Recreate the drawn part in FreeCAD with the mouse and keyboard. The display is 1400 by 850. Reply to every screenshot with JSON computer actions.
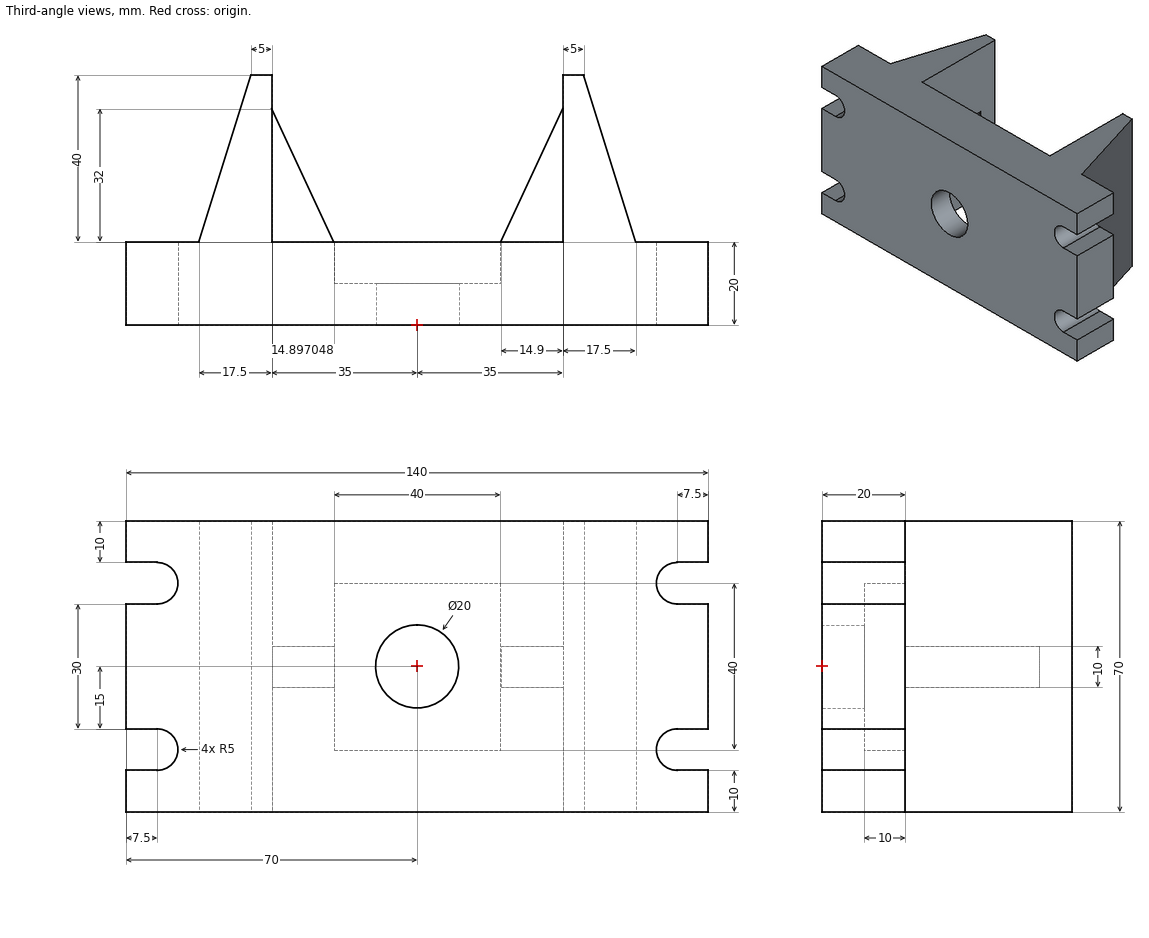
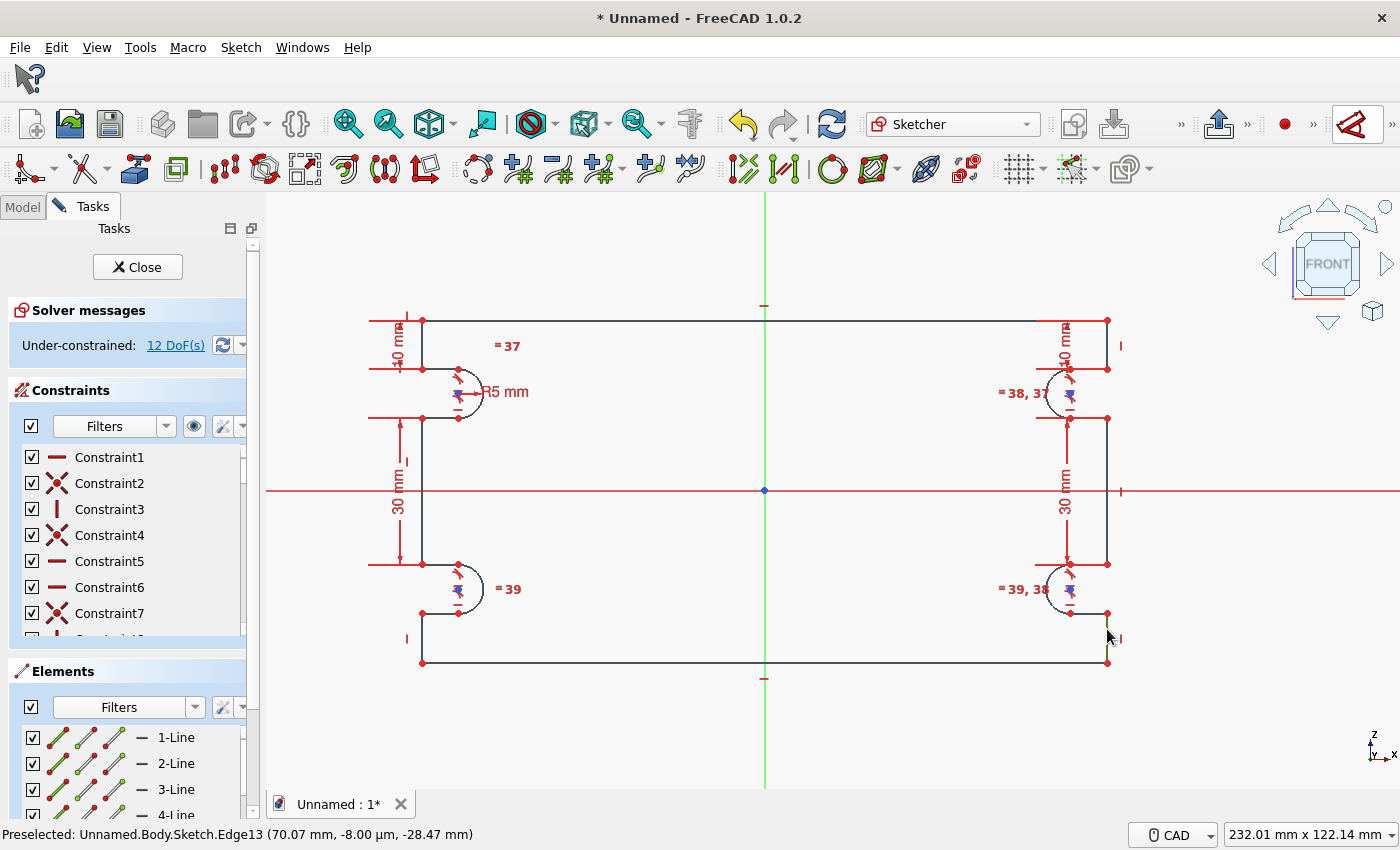
{"action": "key", "text": "i"}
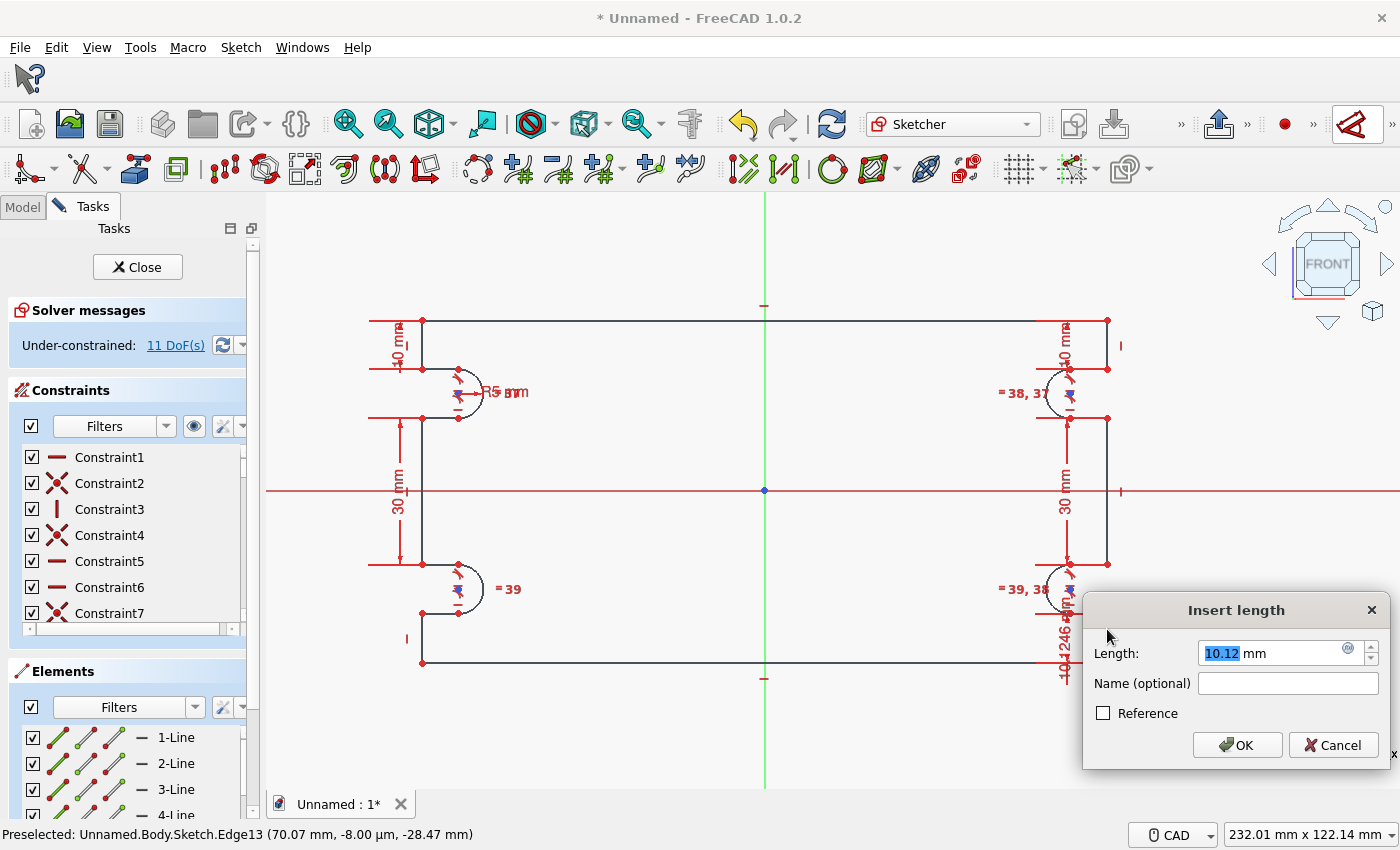
{"action": "type", "text": "10"}
{"action": "key", "text": "Return"}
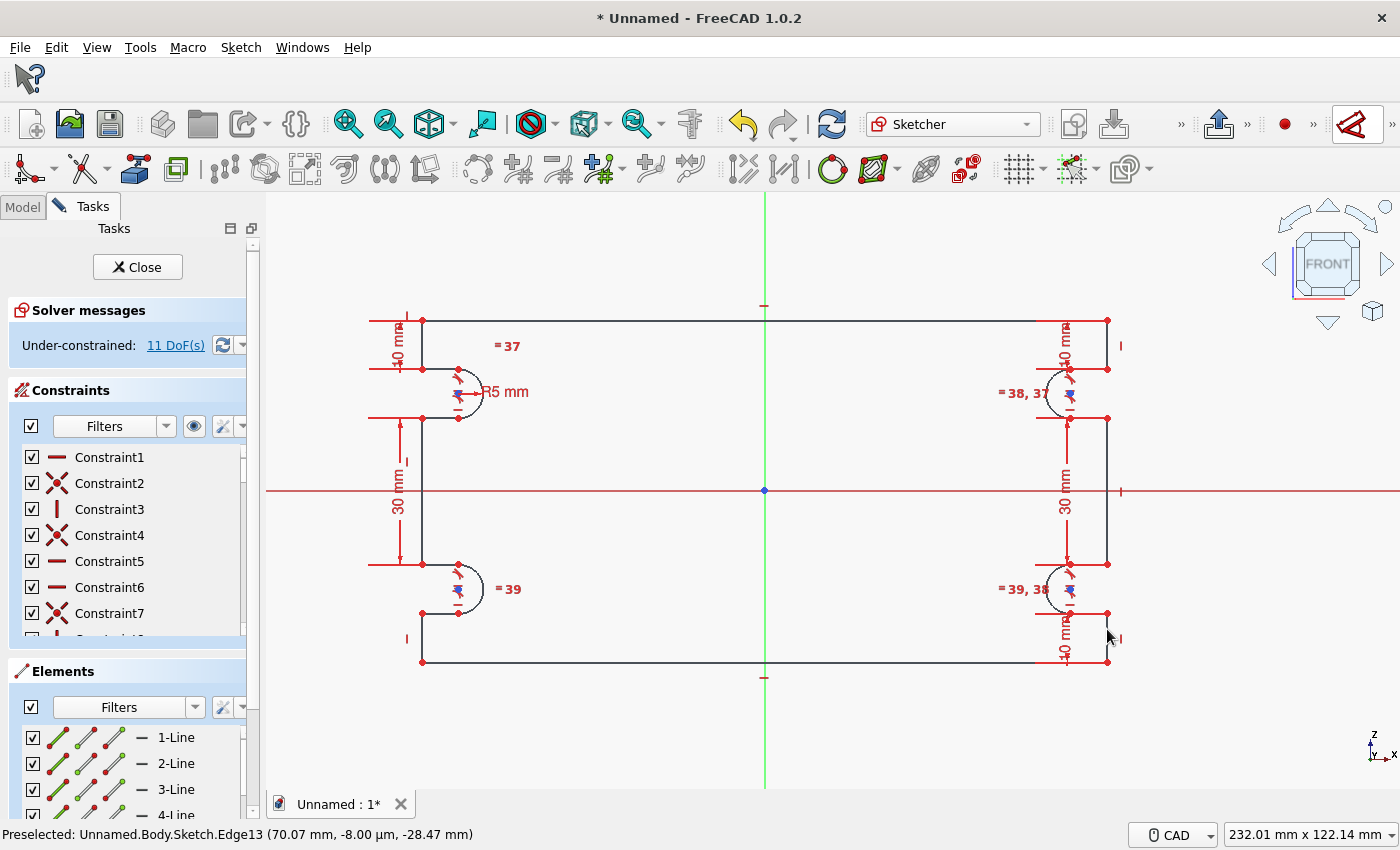
{"action": "scroll", "coordinate": [448, 565], "scroll_direction": "up", "scroll_amount": 2}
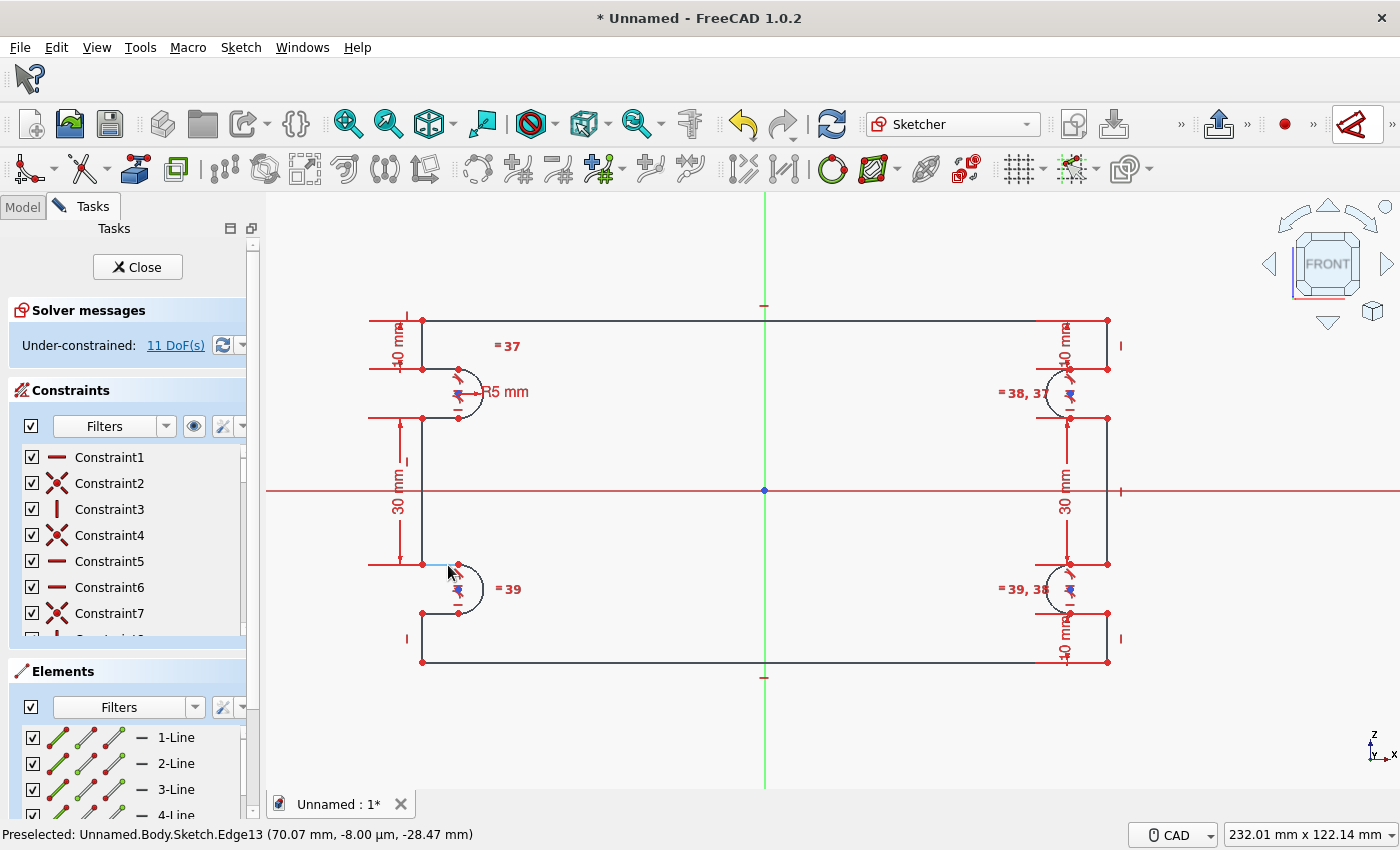
{"action": "left_click", "coordinate": [448, 565]}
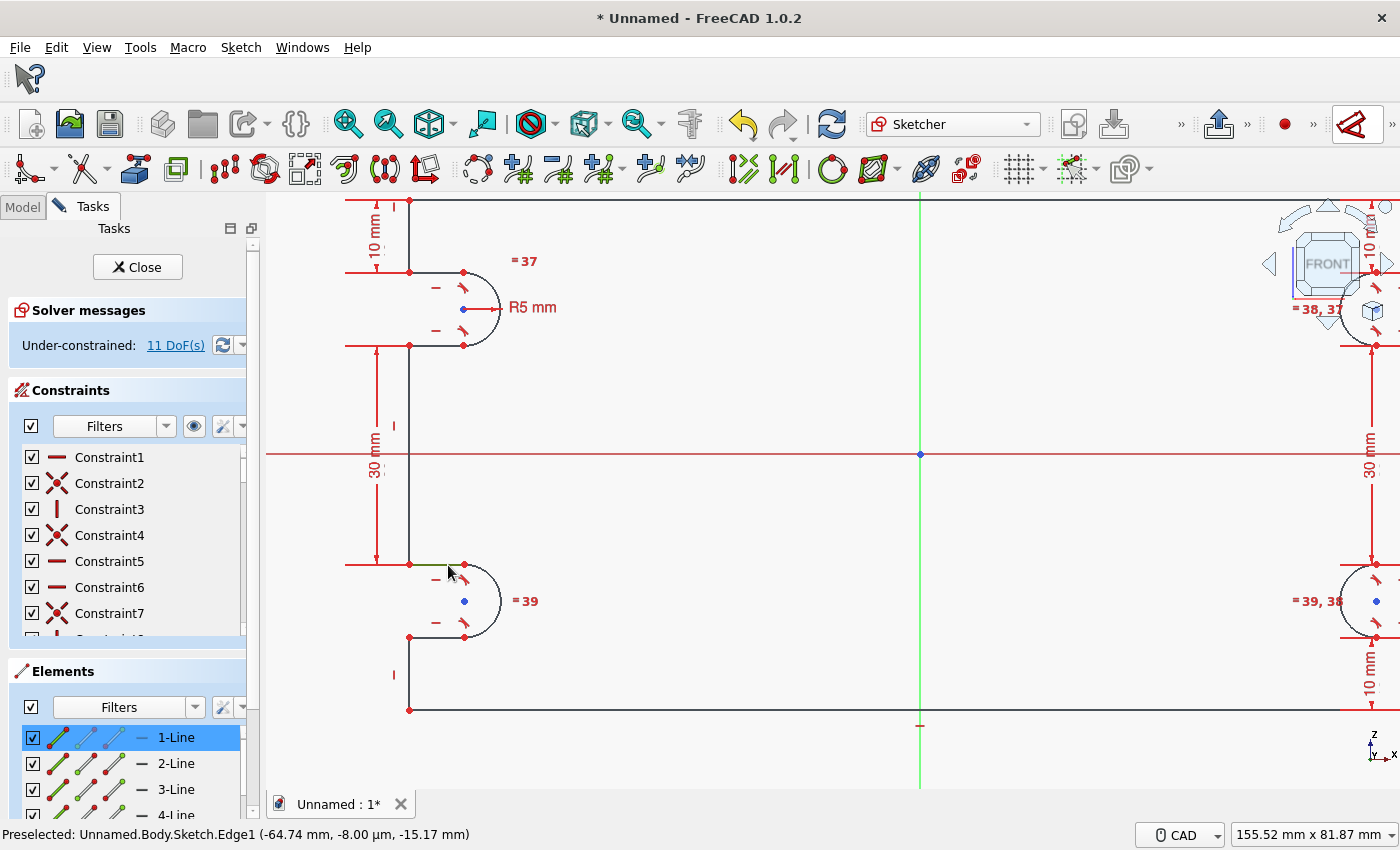
{"action": "key", "text": "l"}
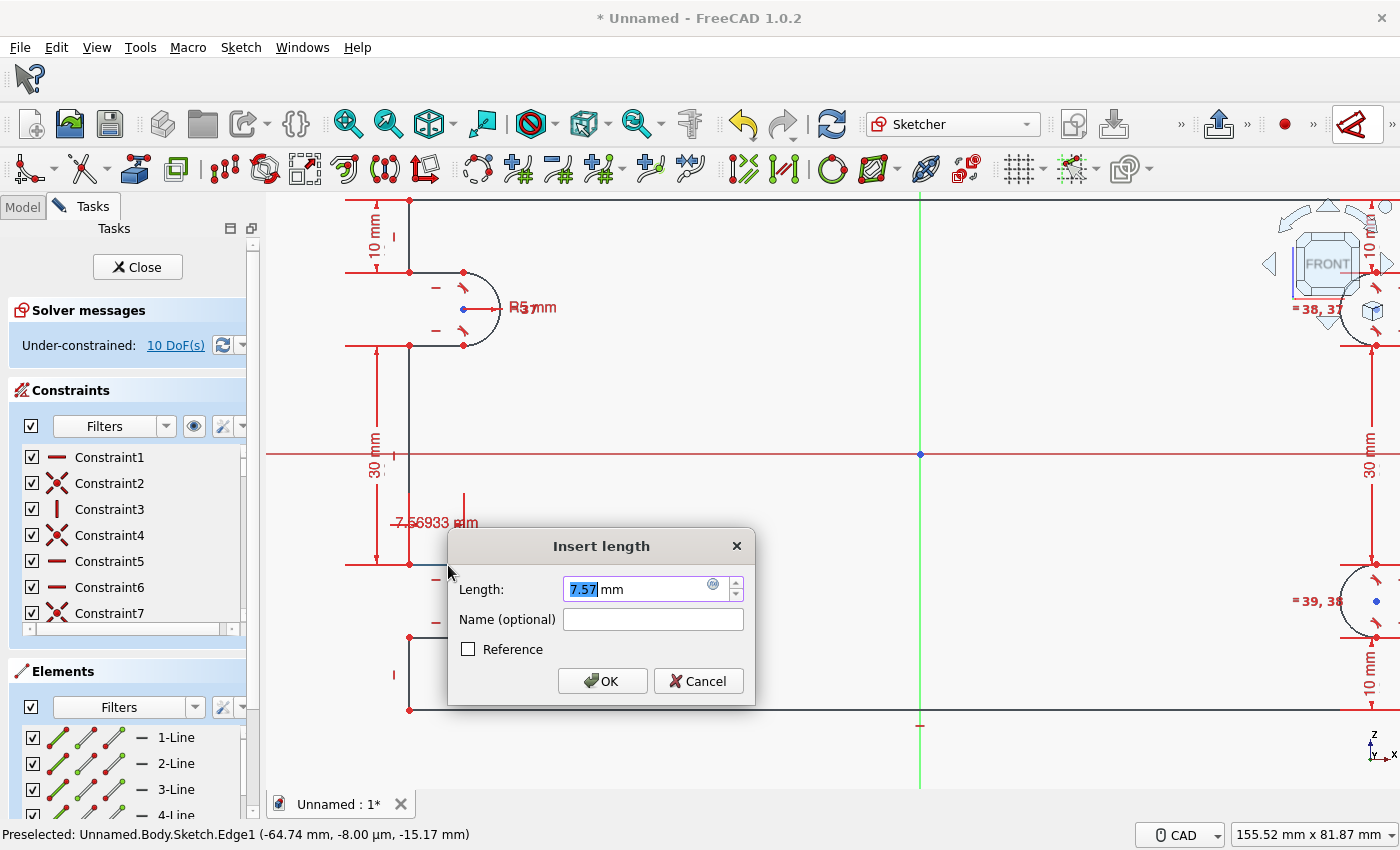
{"action": "type", "text": "7.5"}
{"action": "key", "text": "Return"}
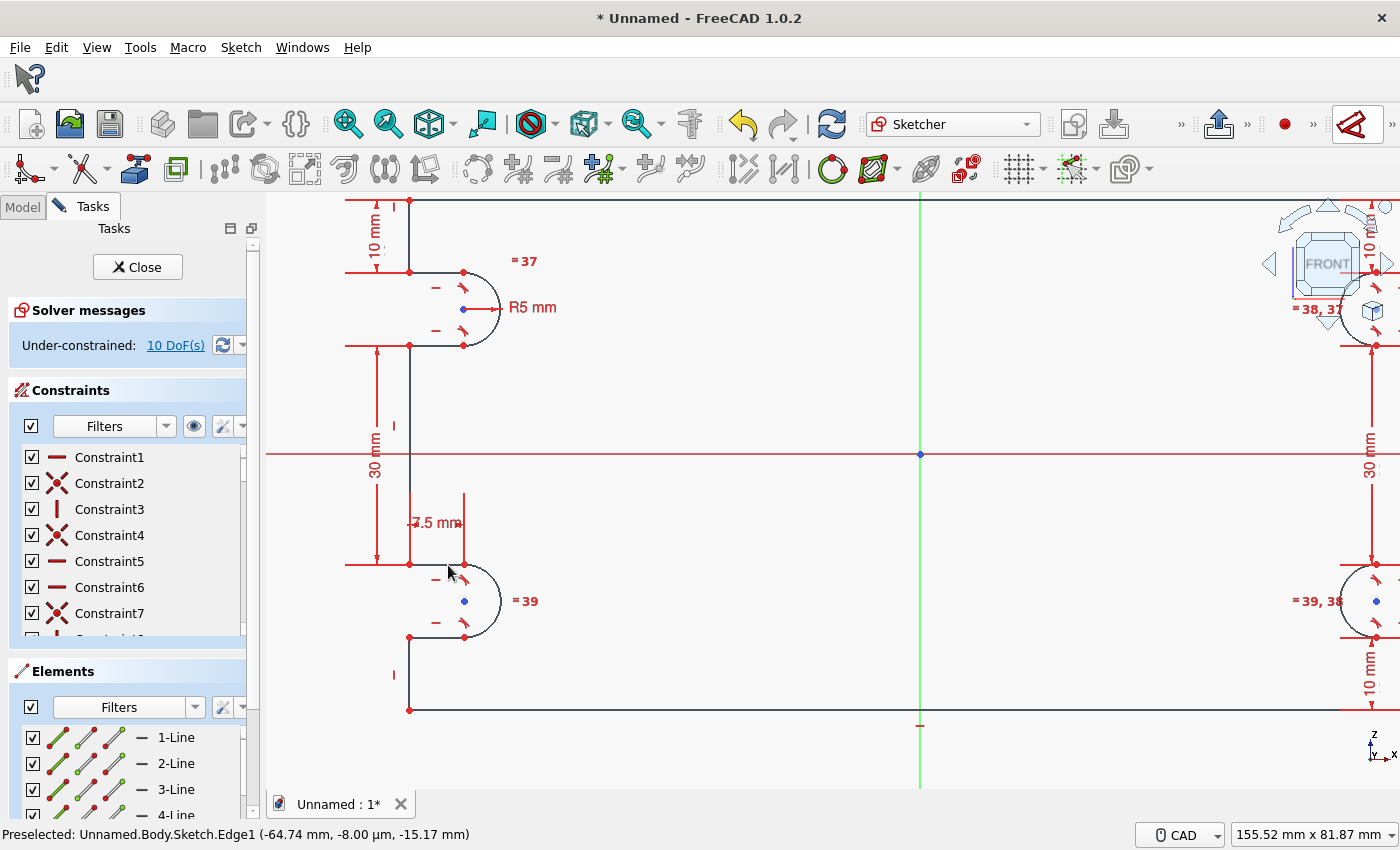
{"action": "left_click", "coordinate": [426, 346]}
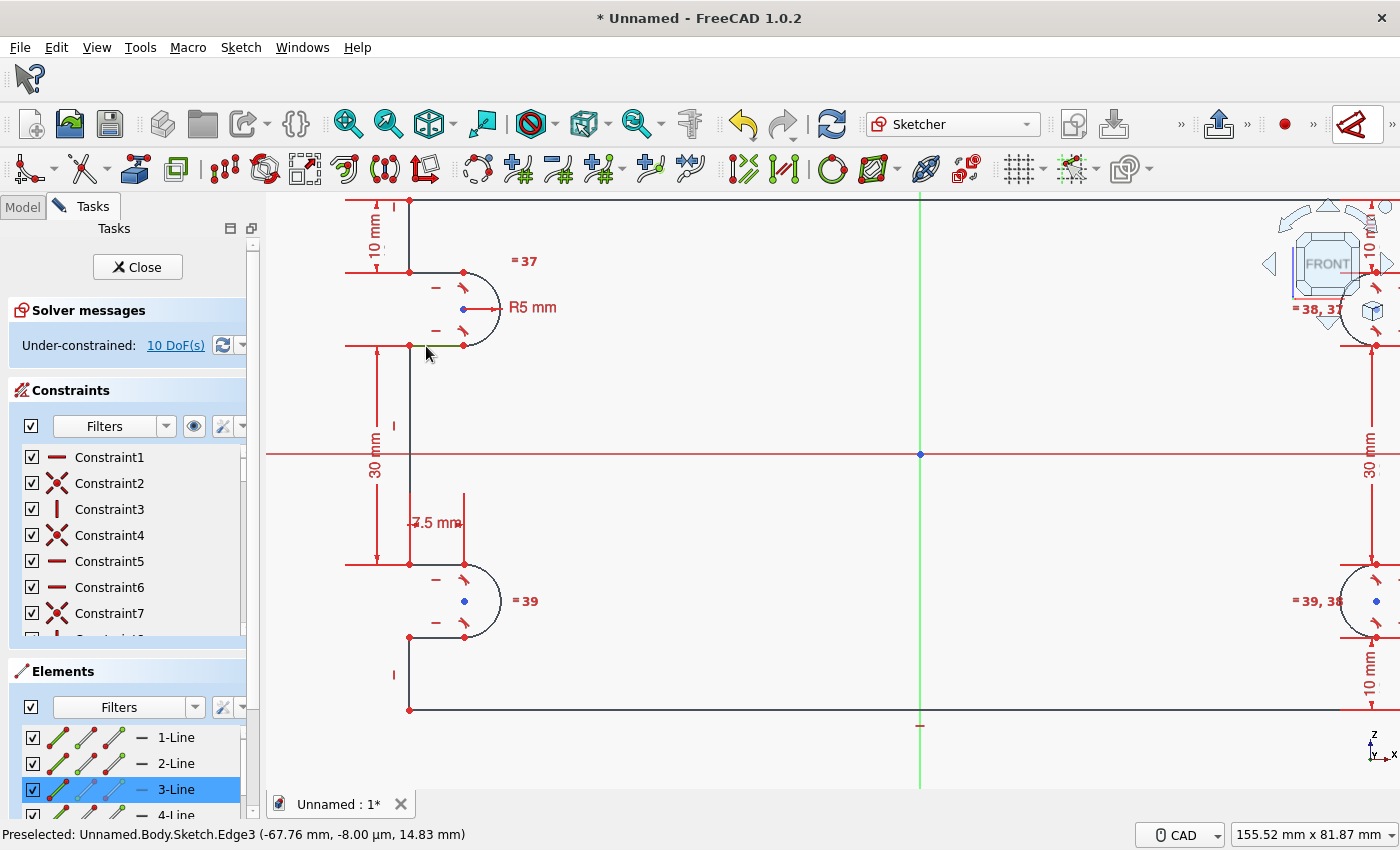
{"action": "key", "text": "l"}